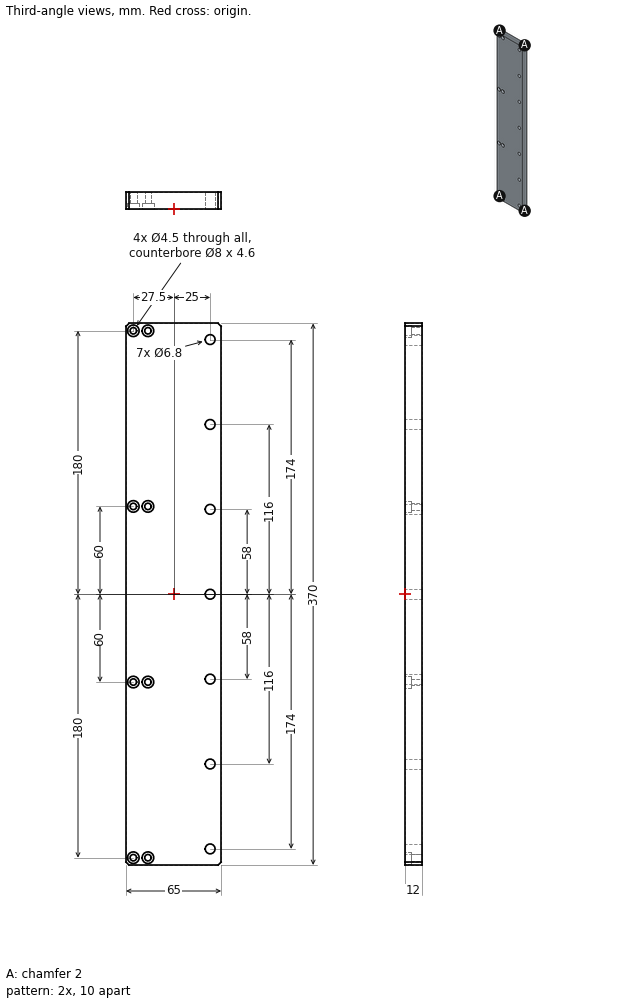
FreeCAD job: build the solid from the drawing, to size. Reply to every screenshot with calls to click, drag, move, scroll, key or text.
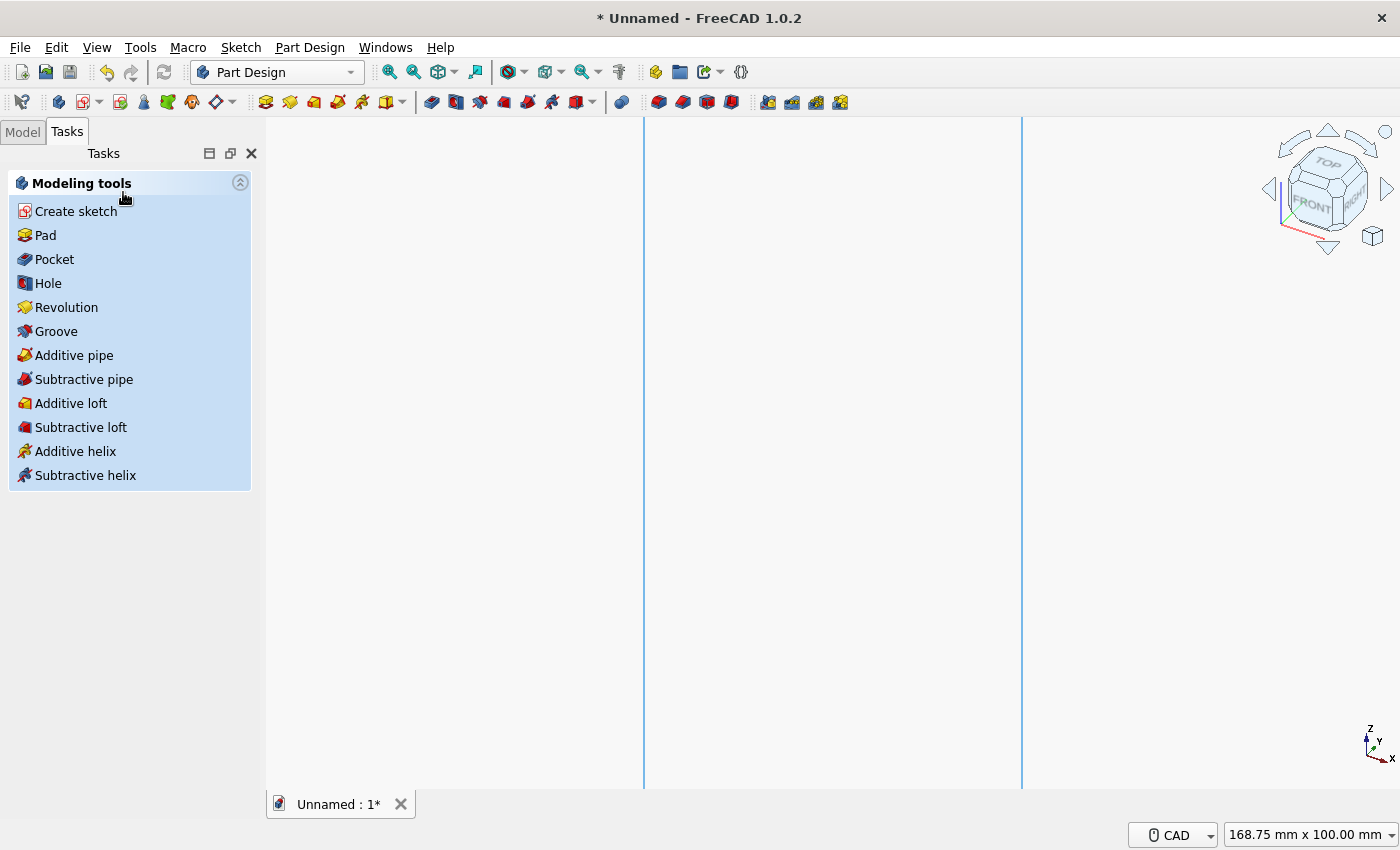
click(266, 102)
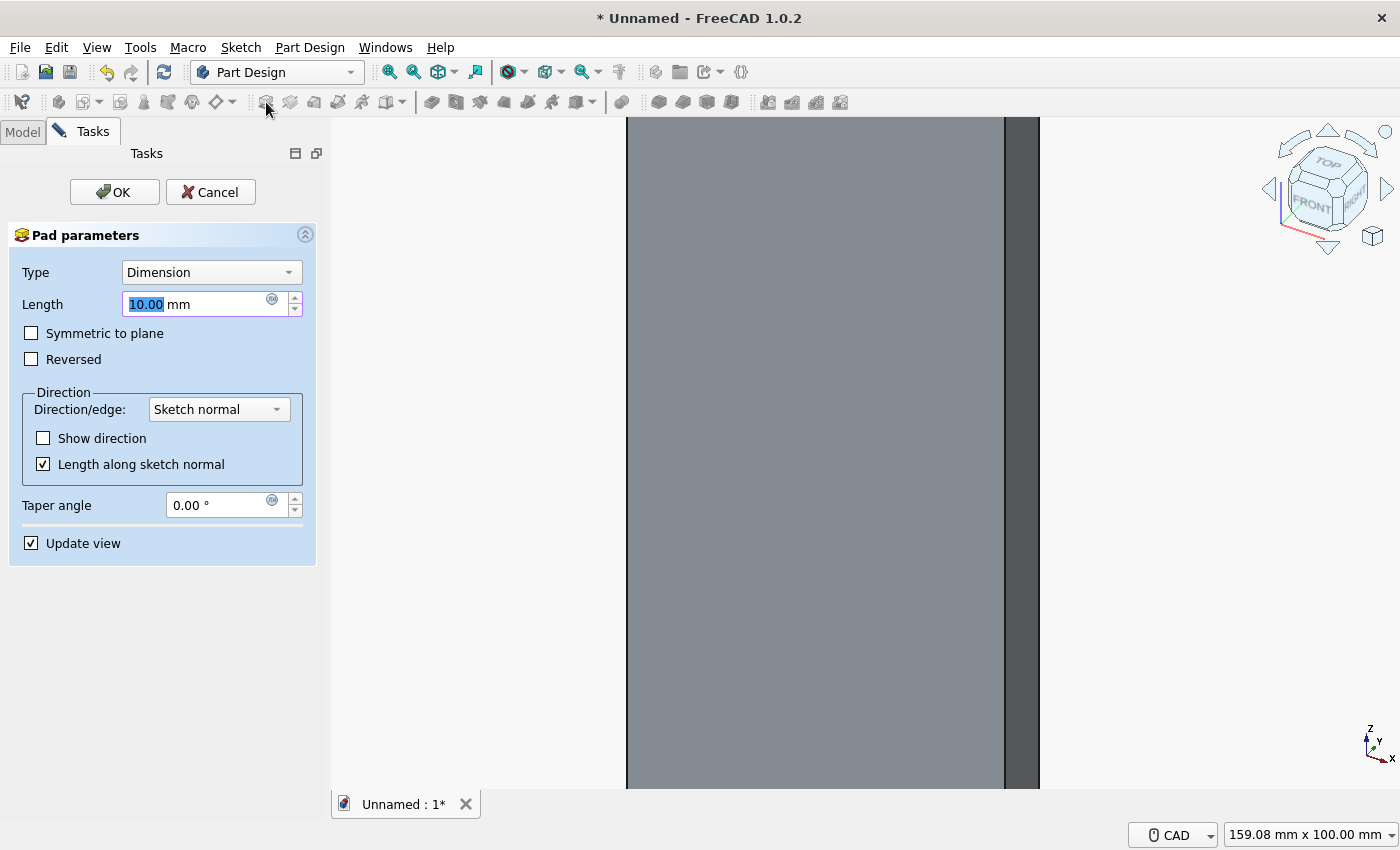
text(12)
key(Tab)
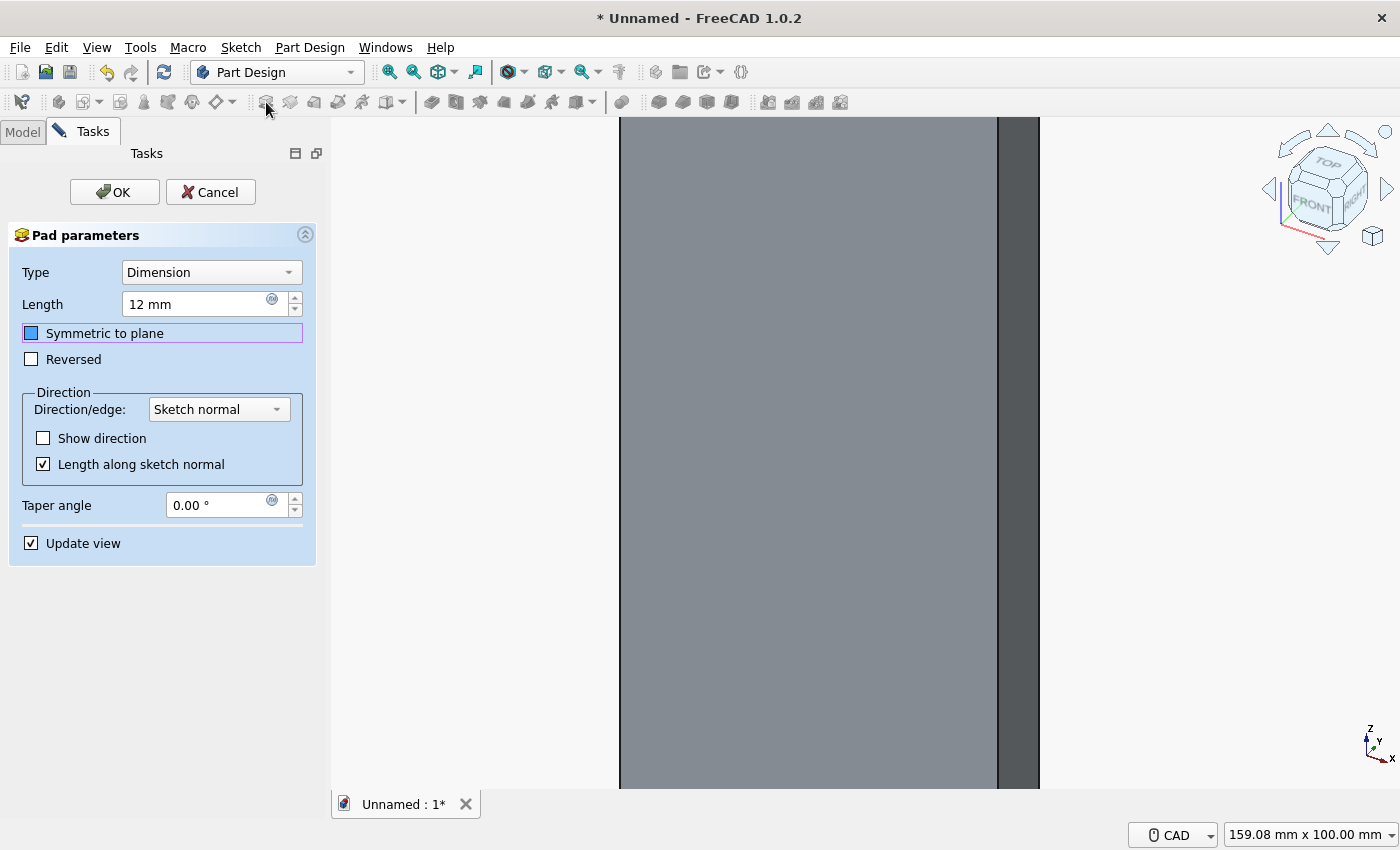
click(30, 359)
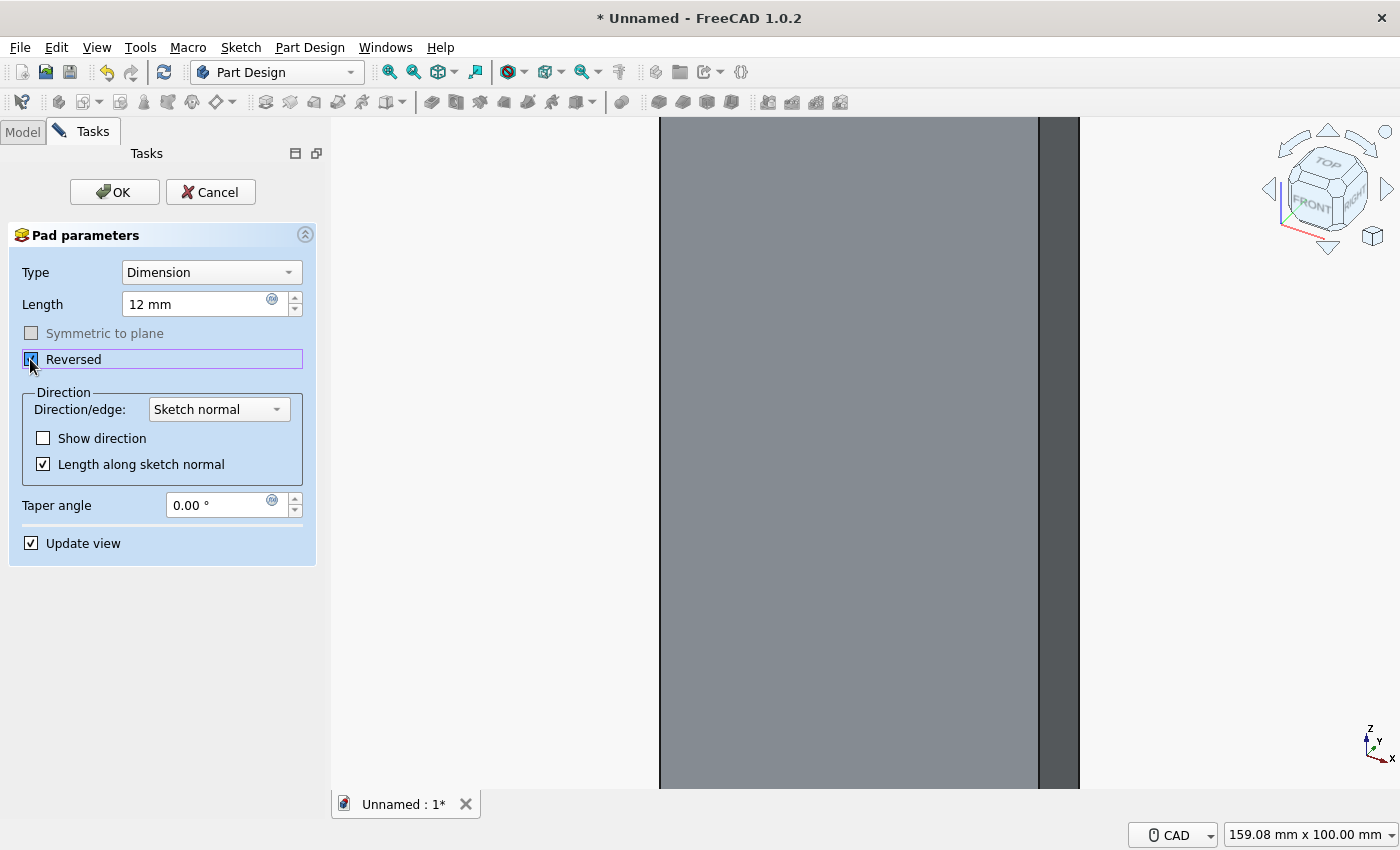
click(115, 192)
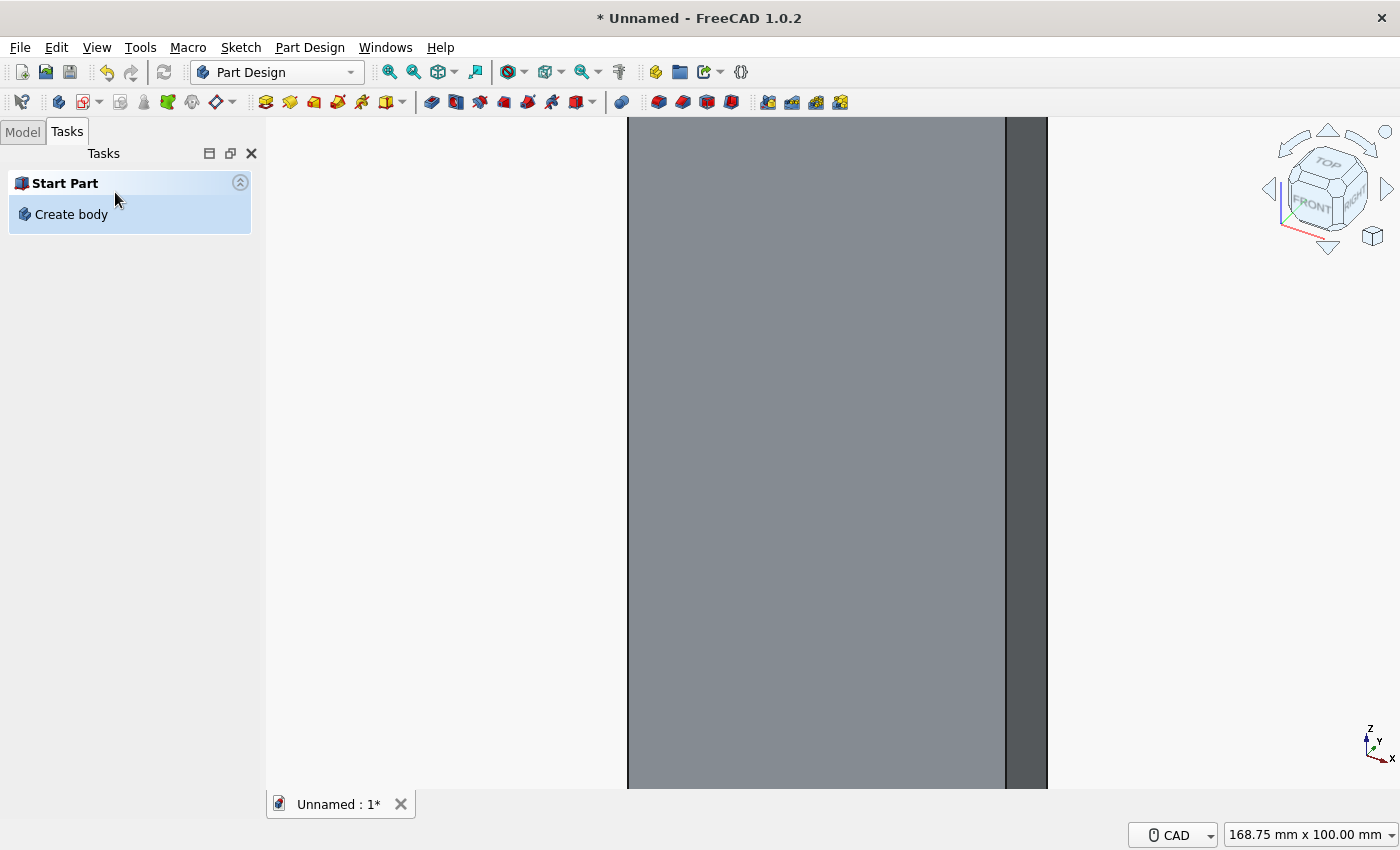
key(v)
key(f)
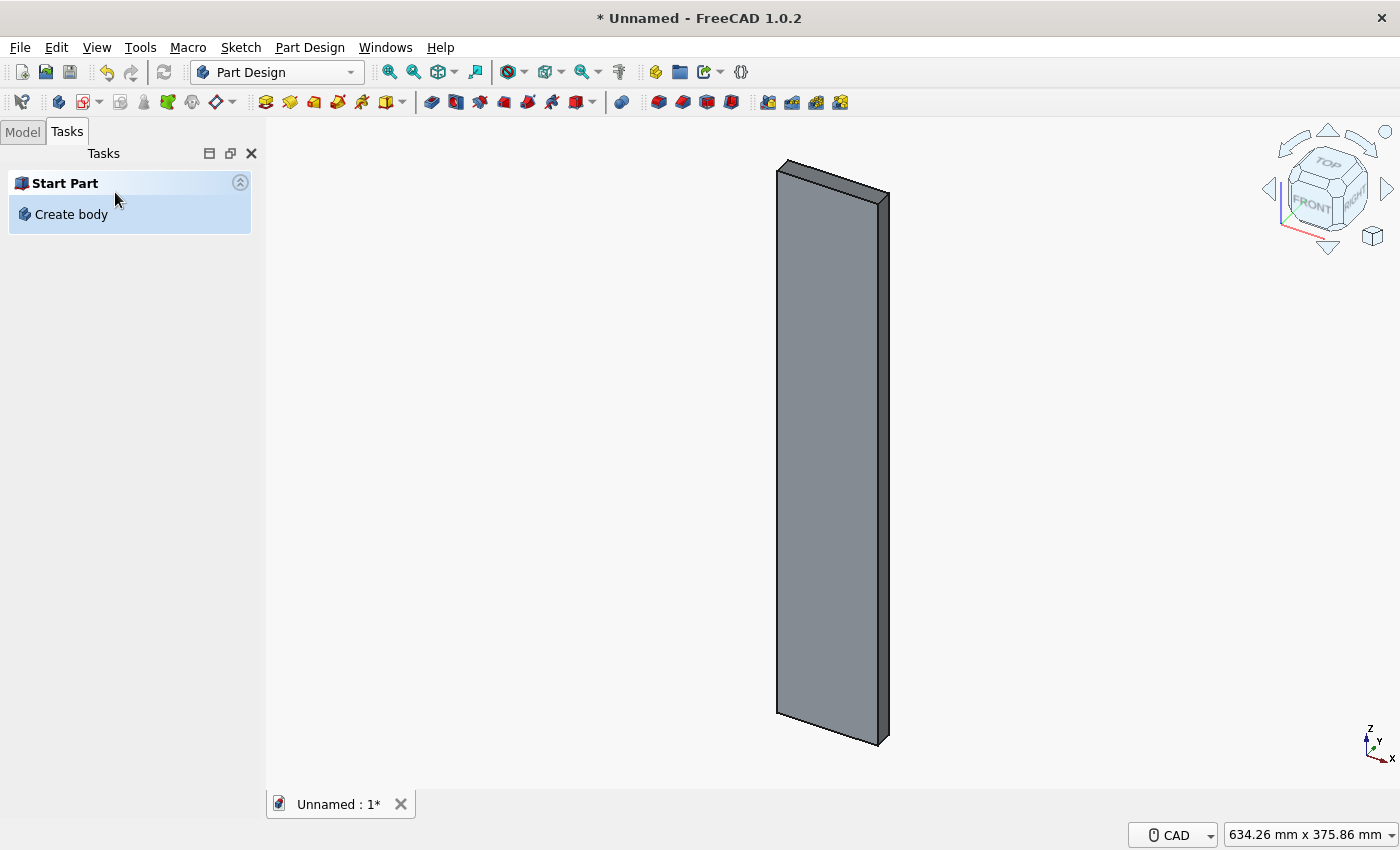
key(4)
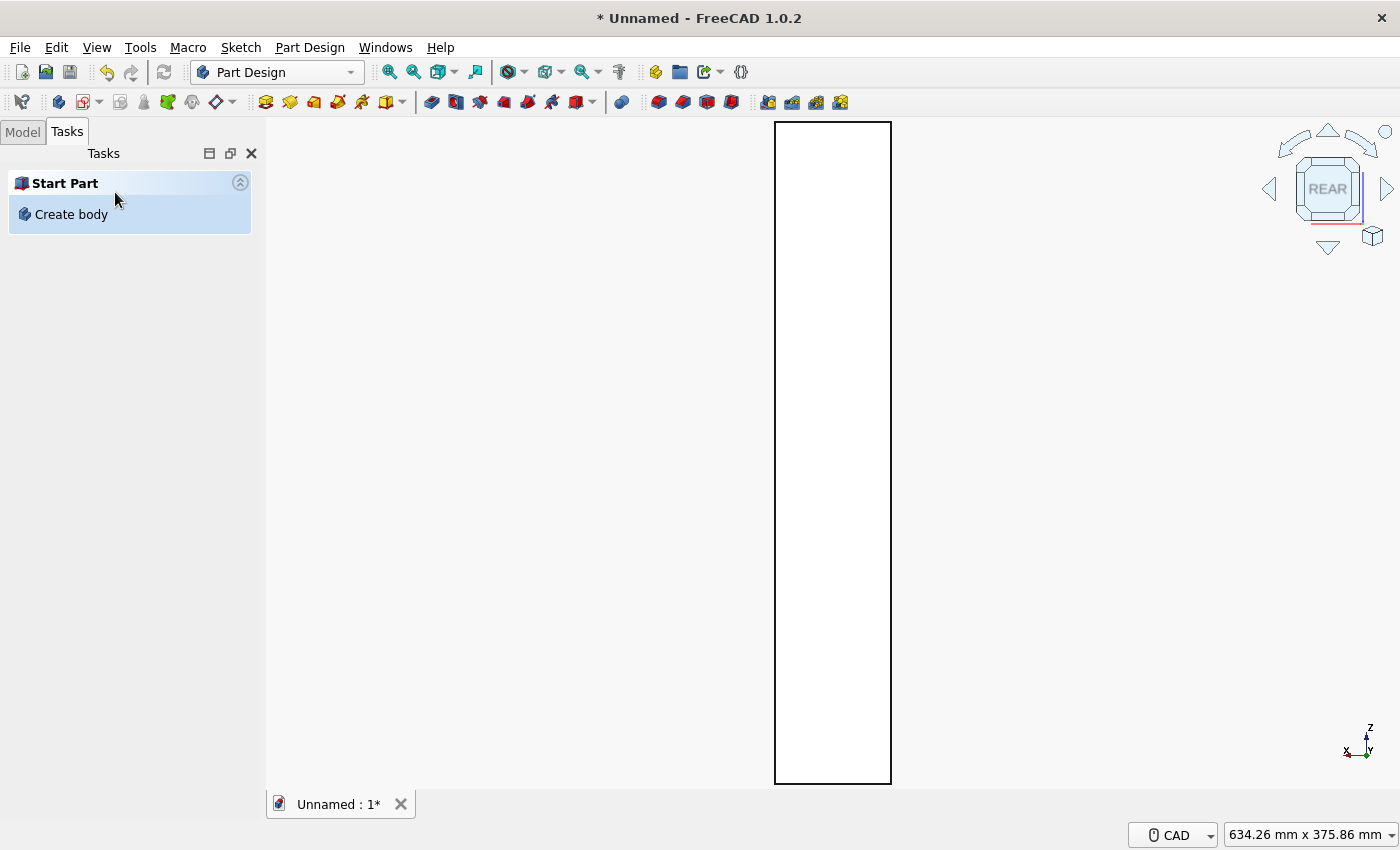
click(833, 263)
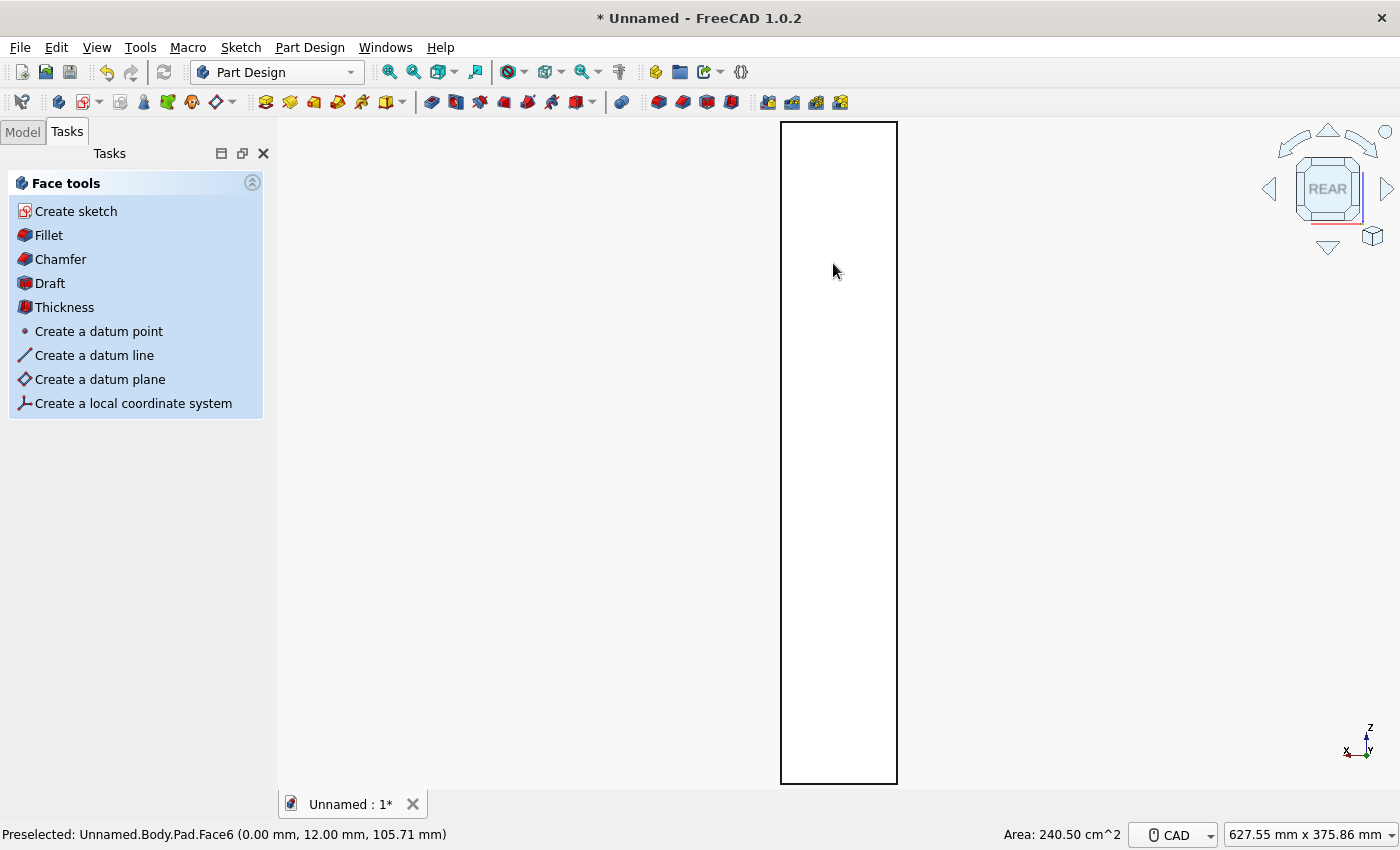
click(84, 102)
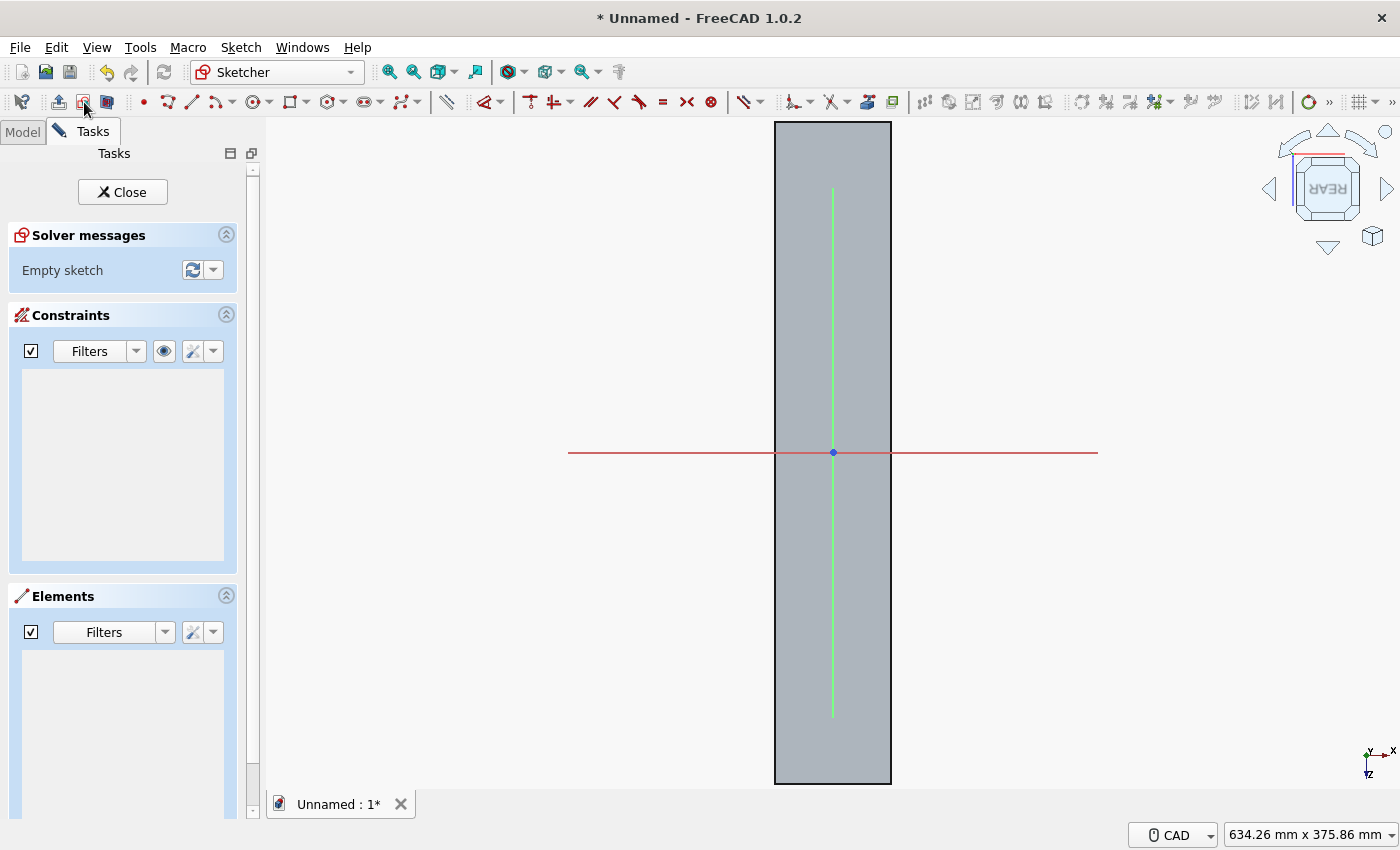
scroll(574, 453, down, 2)